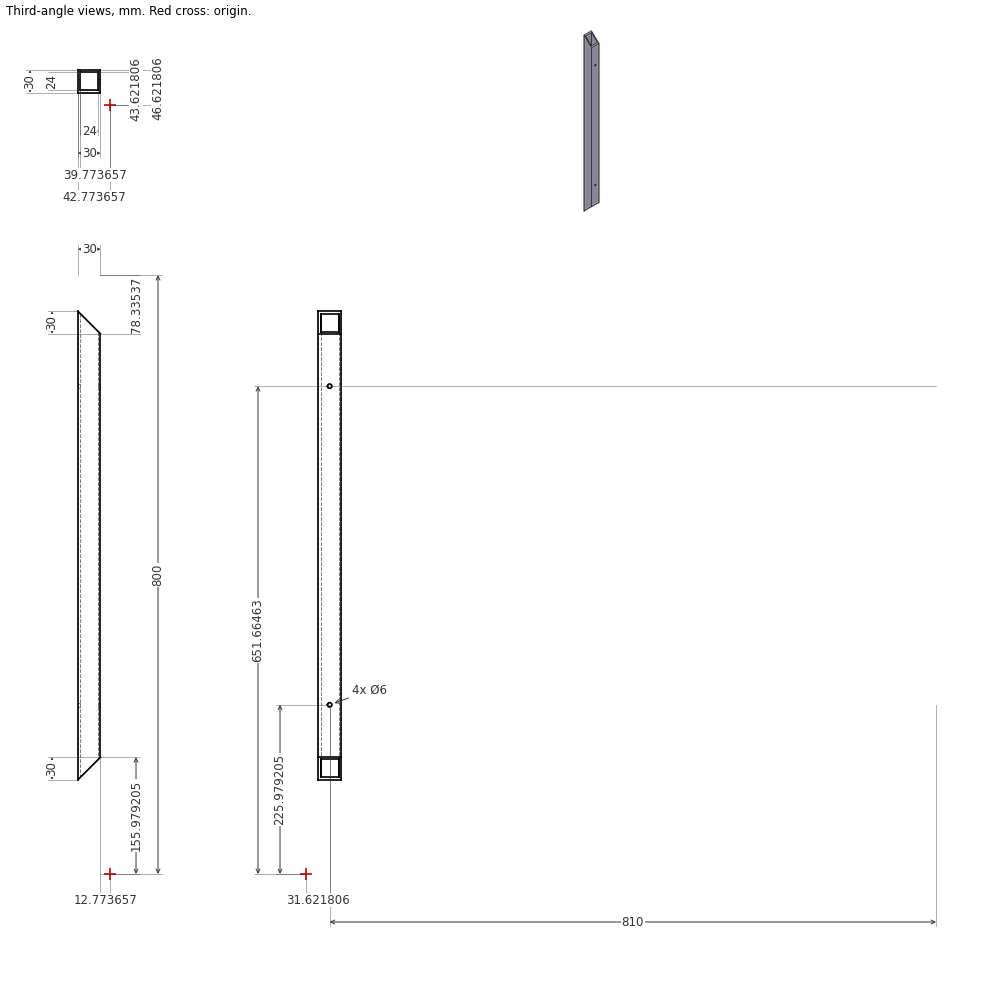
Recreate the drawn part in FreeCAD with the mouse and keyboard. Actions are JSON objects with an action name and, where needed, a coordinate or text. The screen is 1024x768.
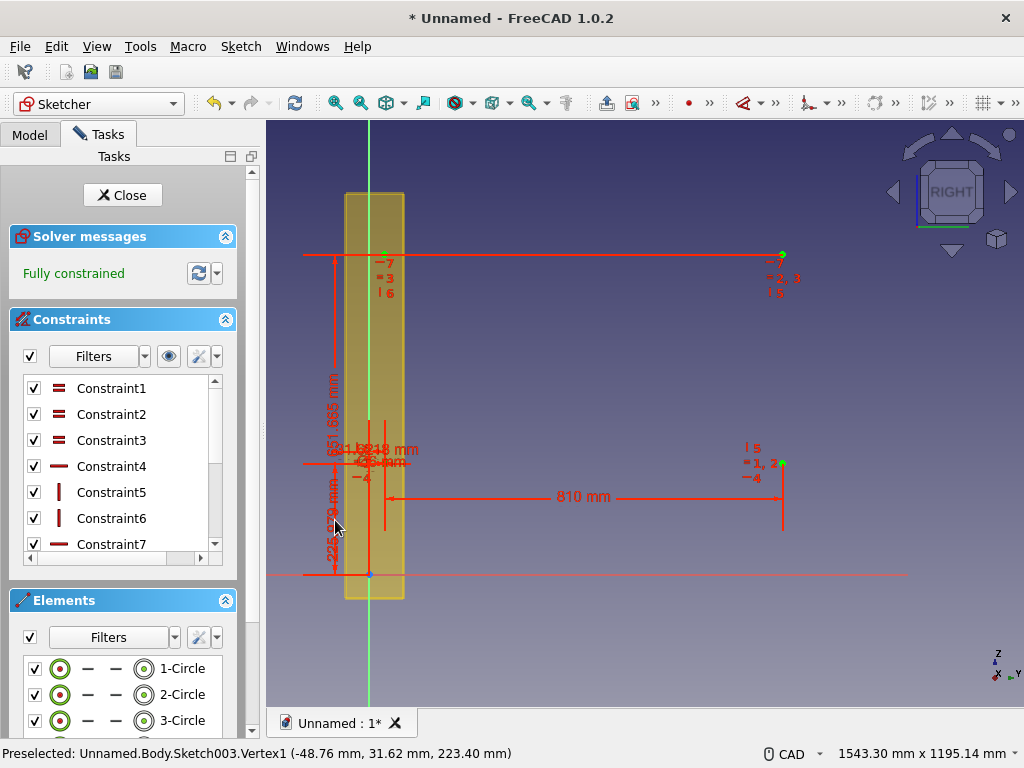
{"action": "left_click", "coordinate": [123, 195]}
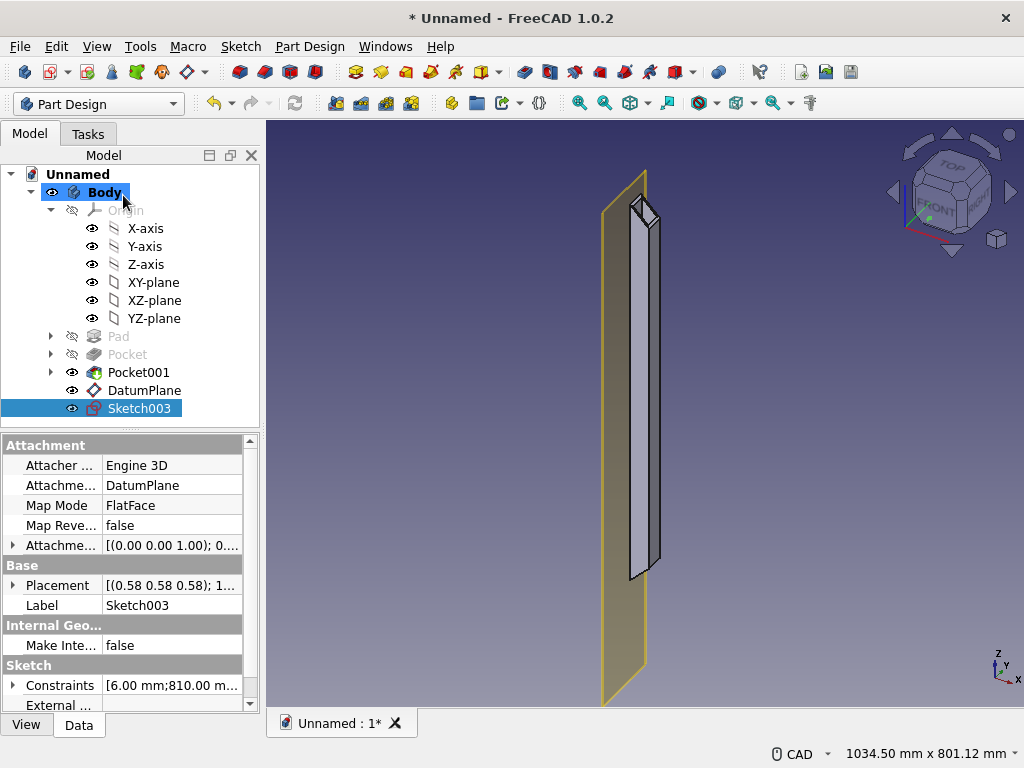
{"action": "left_click", "coordinate": [525, 72]}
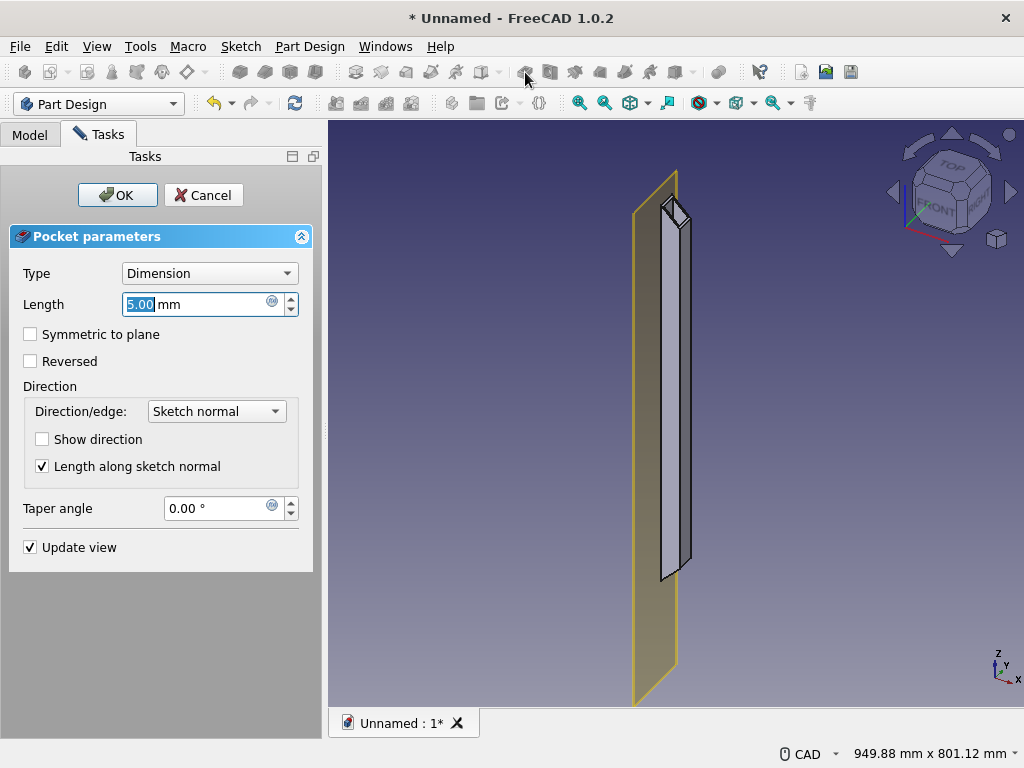
{"action": "left_click", "coordinate": [210, 274]}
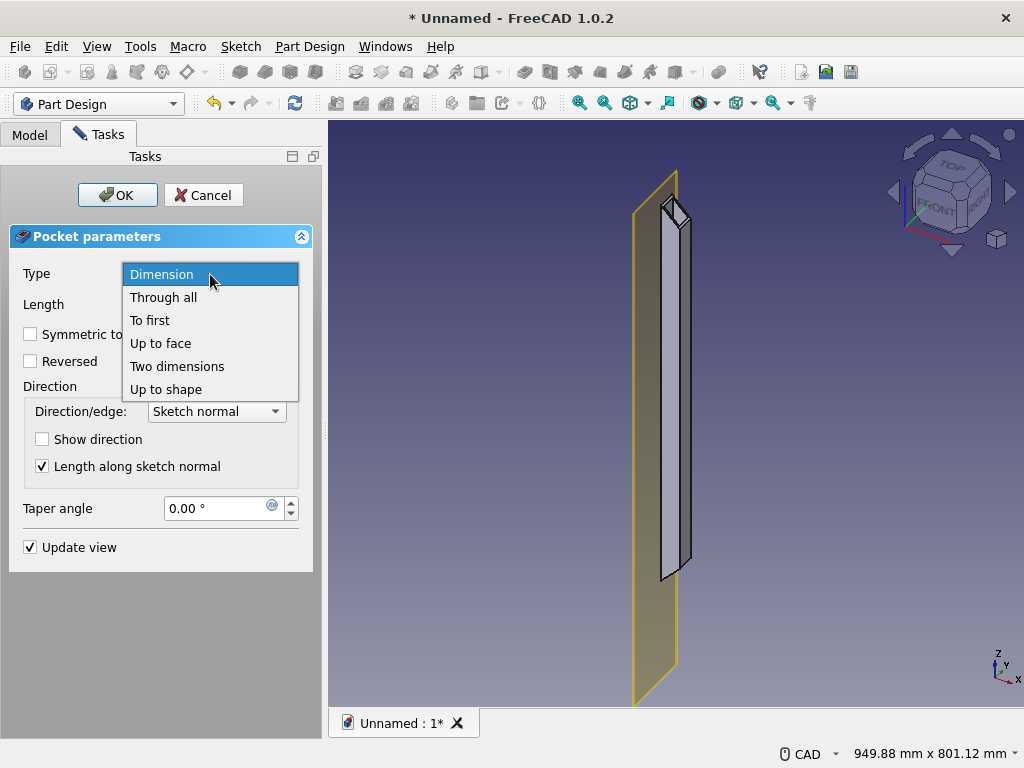
{"action": "left_click", "coordinate": [208, 298]}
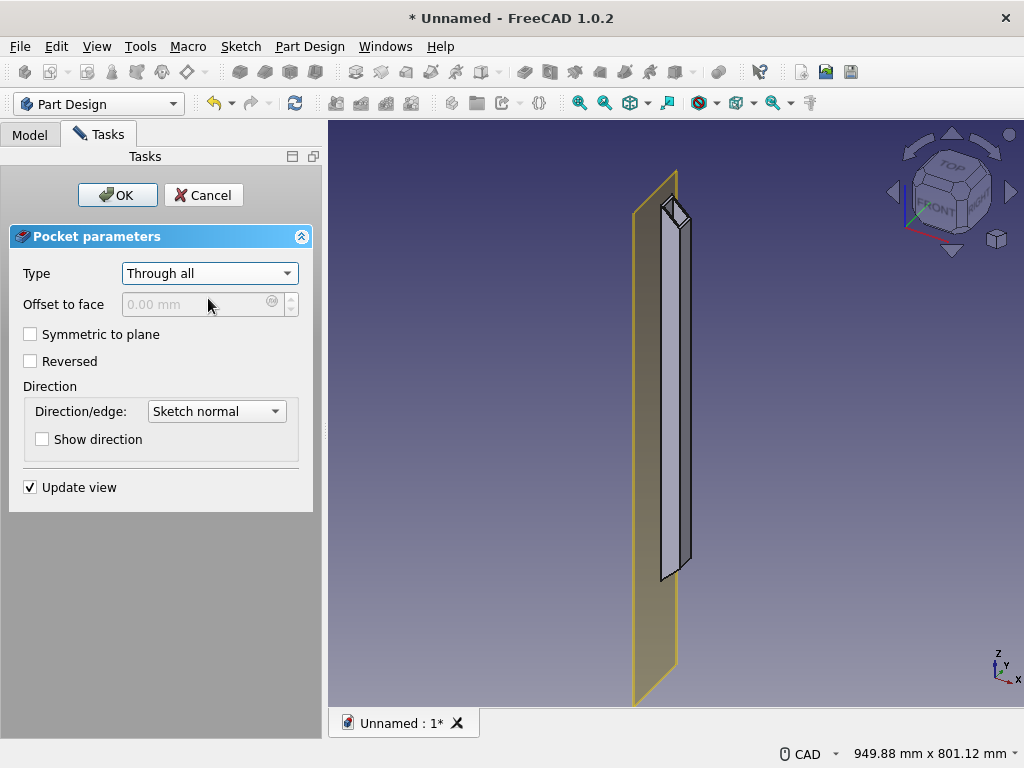
{"action": "left_click", "coordinate": [31, 361]}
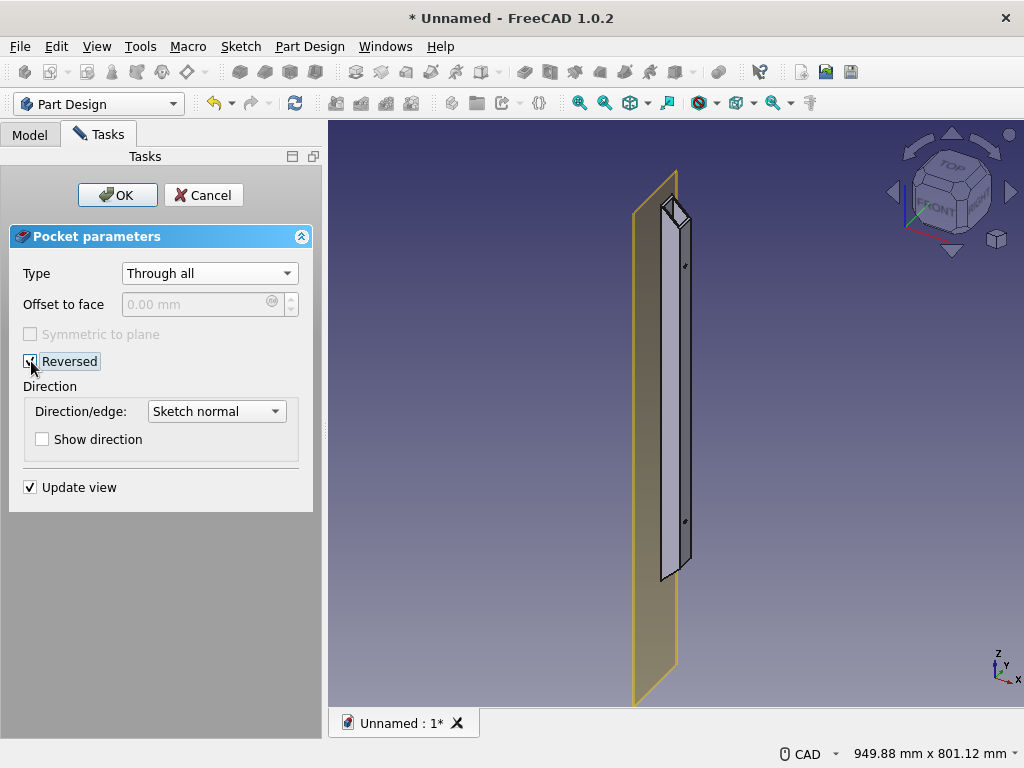
{"action": "left_click", "coordinate": [118, 195]}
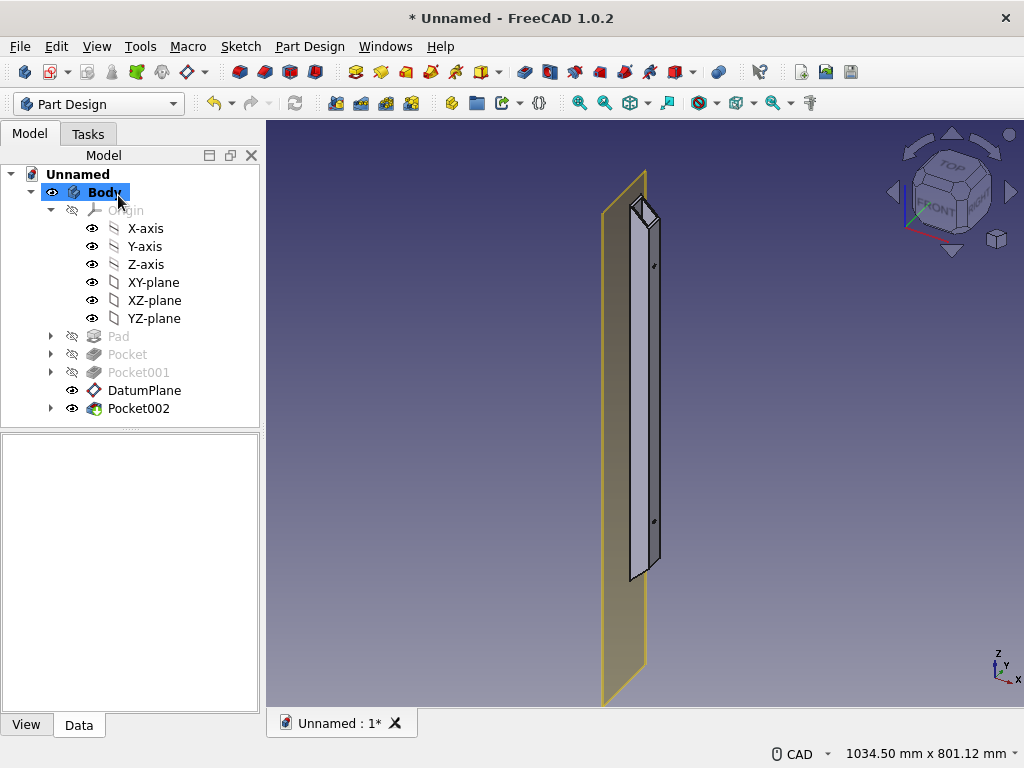
{"action": "left_click", "coordinate": [117, 390]}
{"action": "key", "text": "space"}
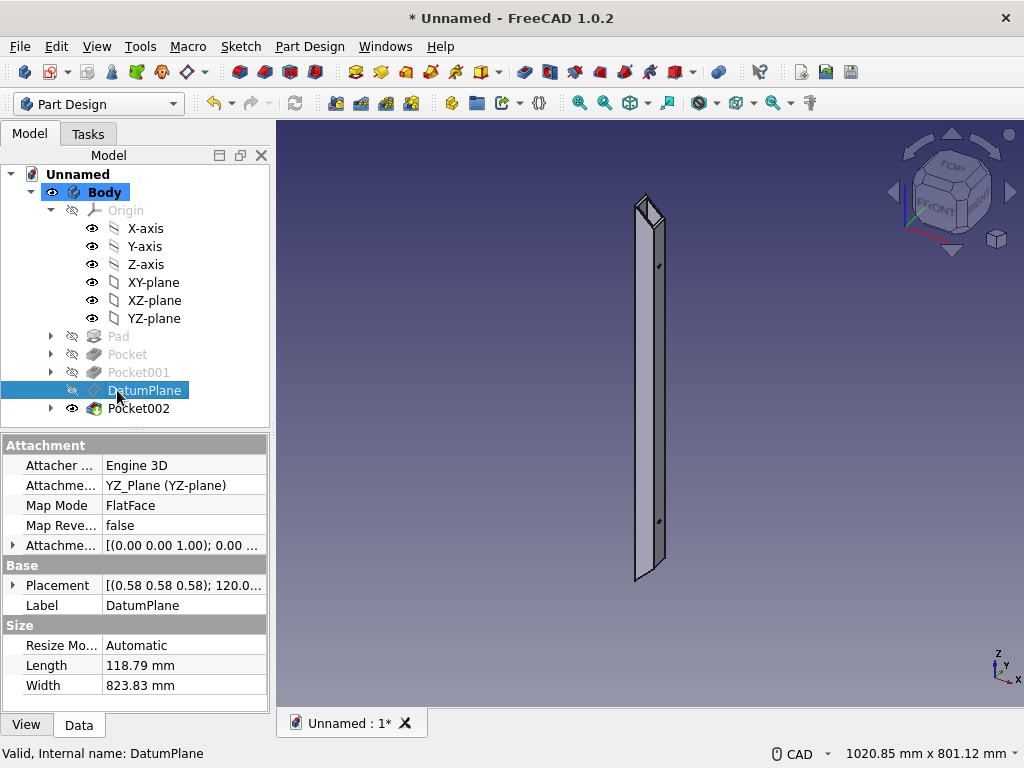
{"action": "key", "text": "0"}